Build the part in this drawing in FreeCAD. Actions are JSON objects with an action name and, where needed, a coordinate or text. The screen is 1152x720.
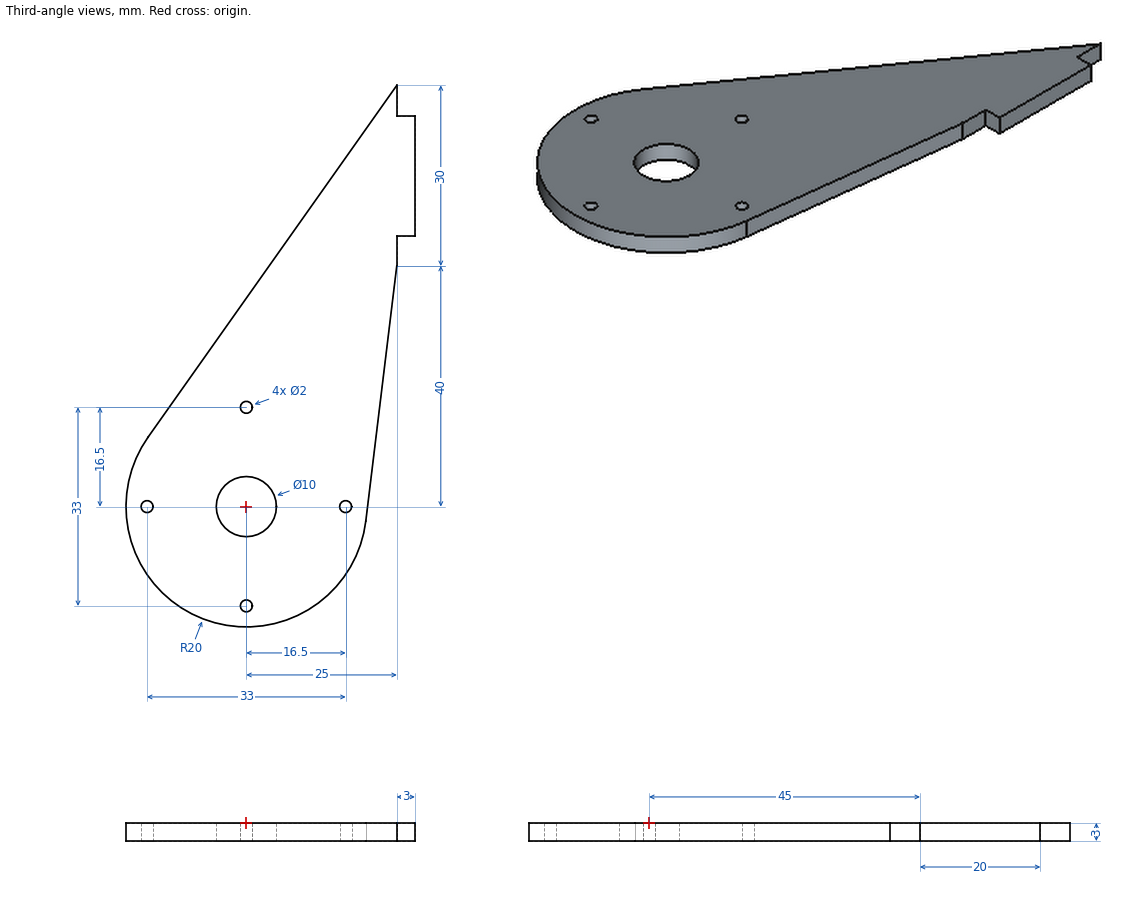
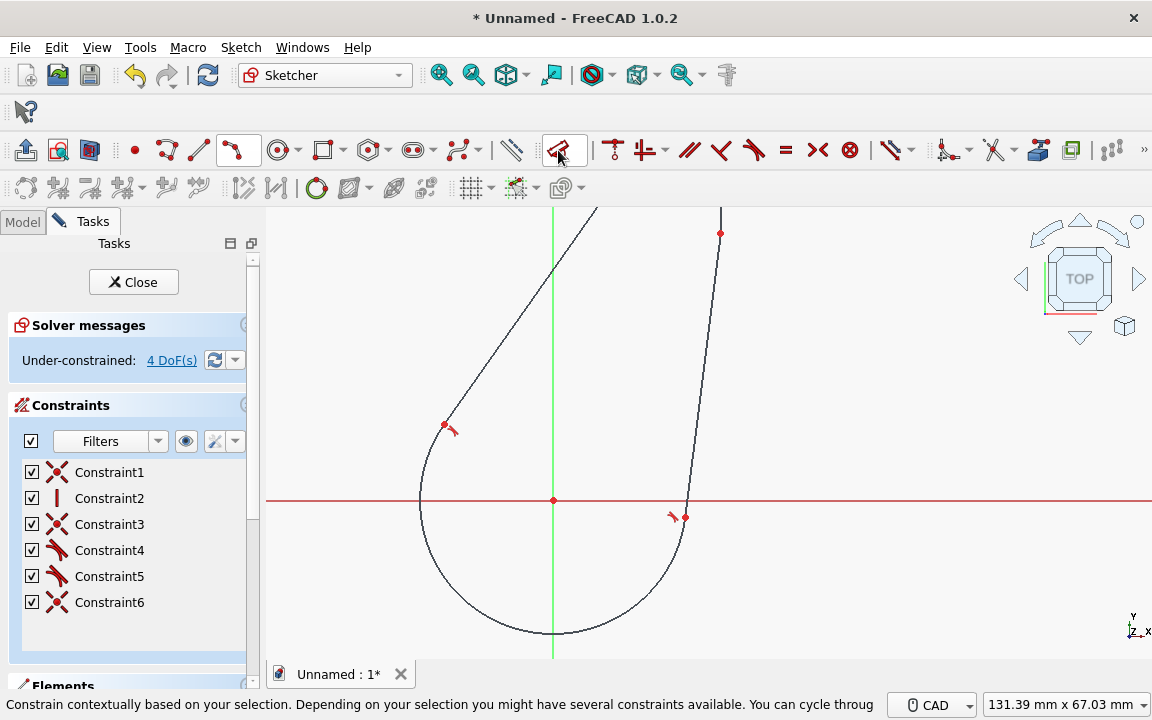
{"action": "left_click", "coordinate": [435, 562]}
{"action": "left_click", "coordinate": [407, 577]}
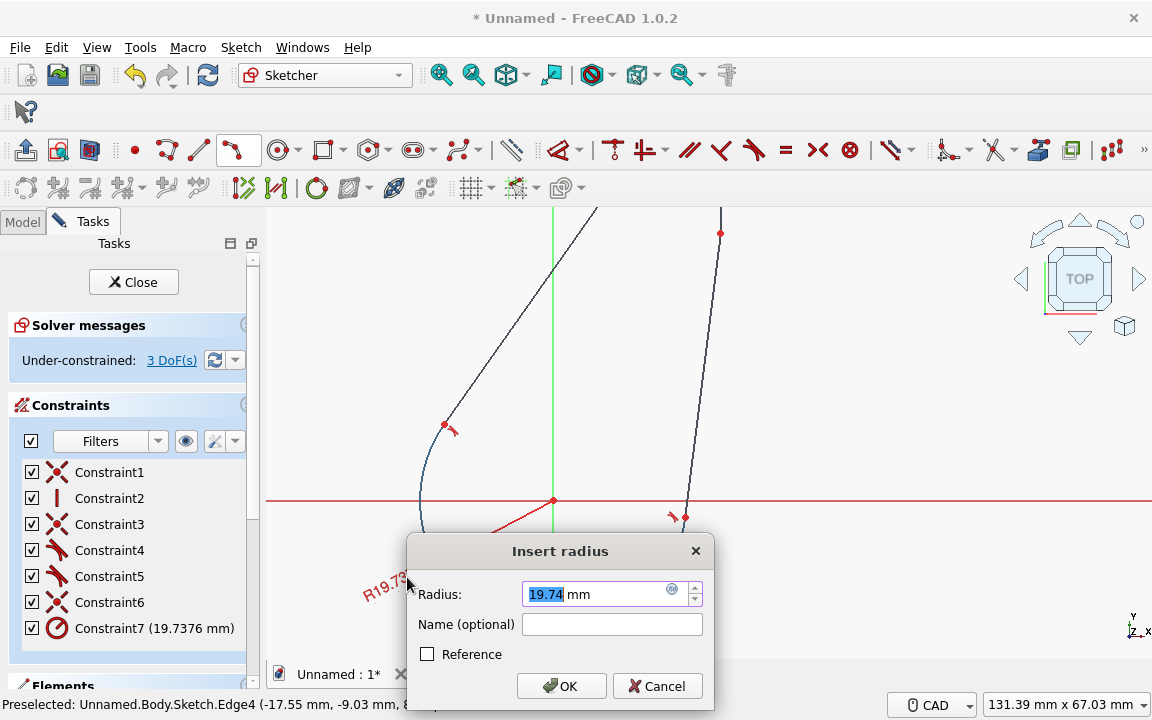
{"action": "type", "text": "20"}
{"action": "key", "text": "Return"}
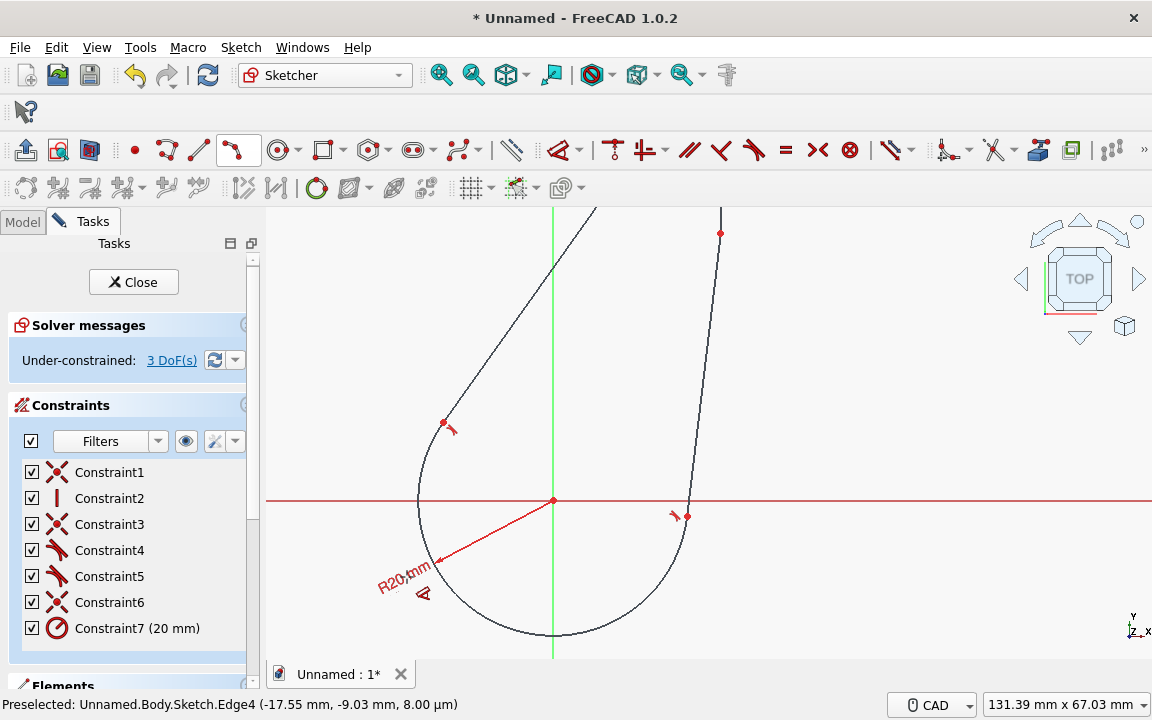
{"action": "scroll", "coordinate": [688, 519], "scroll_direction": "down", "scroll_amount": 4}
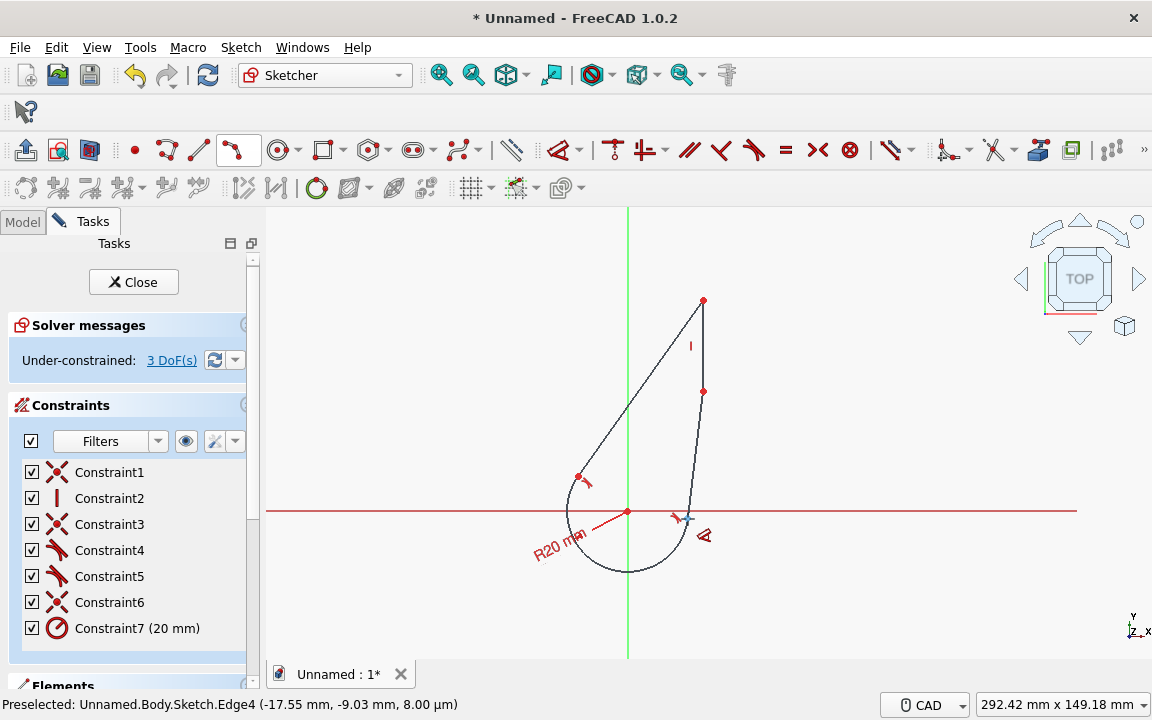
{"action": "left_click", "coordinate": [703, 364]}
{"action": "left_click", "coordinate": [737, 346]}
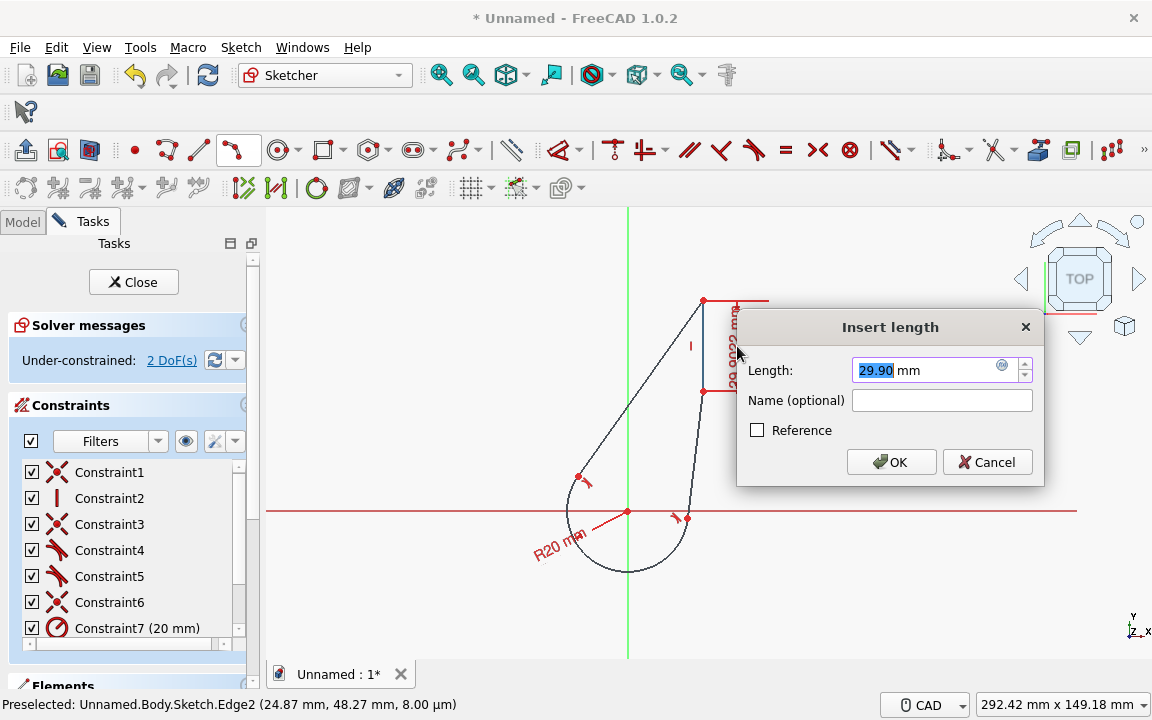
{"action": "type", "text": "30"}
{"action": "key", "text": "Return"}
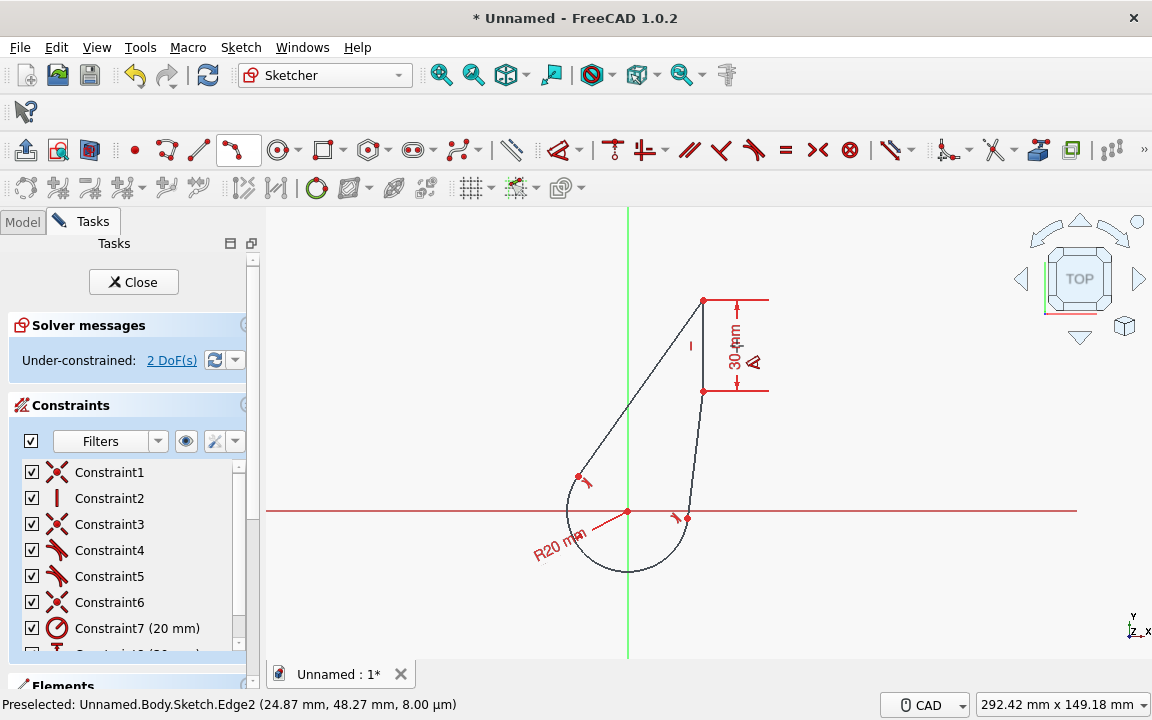
{"action": "left_click", "coordinate": [703, 391]}
{"action": "left_click", "coordinate": [648, 545]}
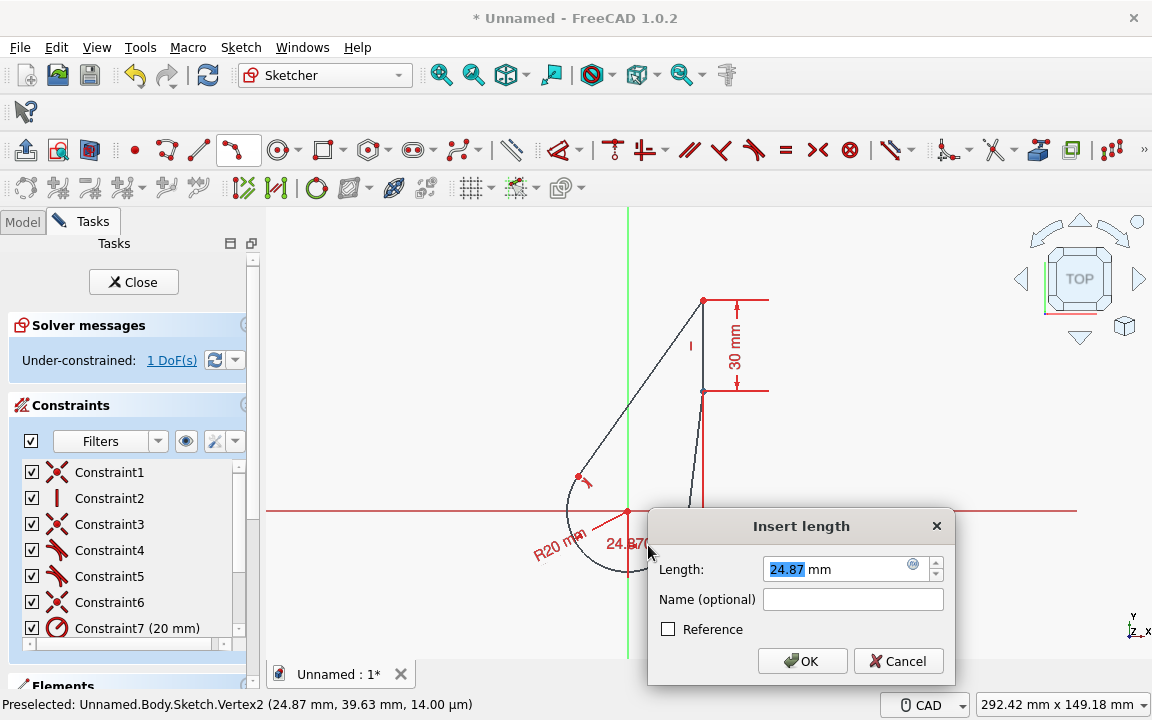
{"action": "type", "text": "25"}
{"action": "key", "text": "Return"}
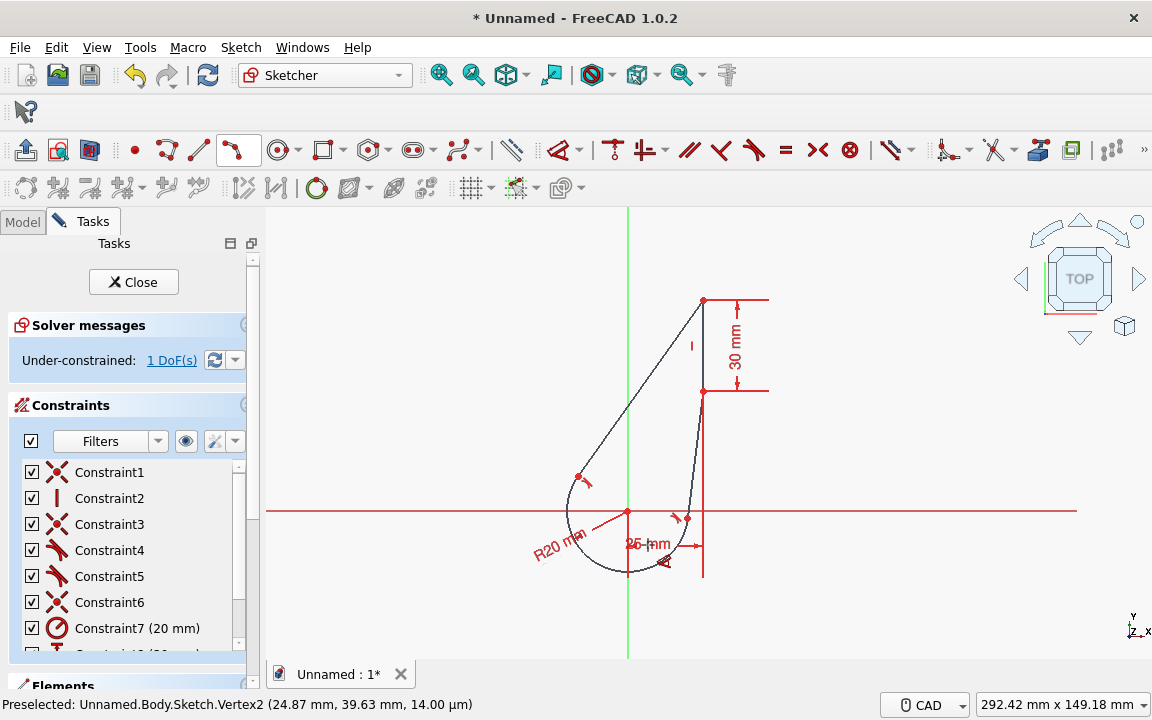
{"action": "left_click", "coordinate": [703, 391]}
{"action": "left_click", "coordinate": [737, 451]}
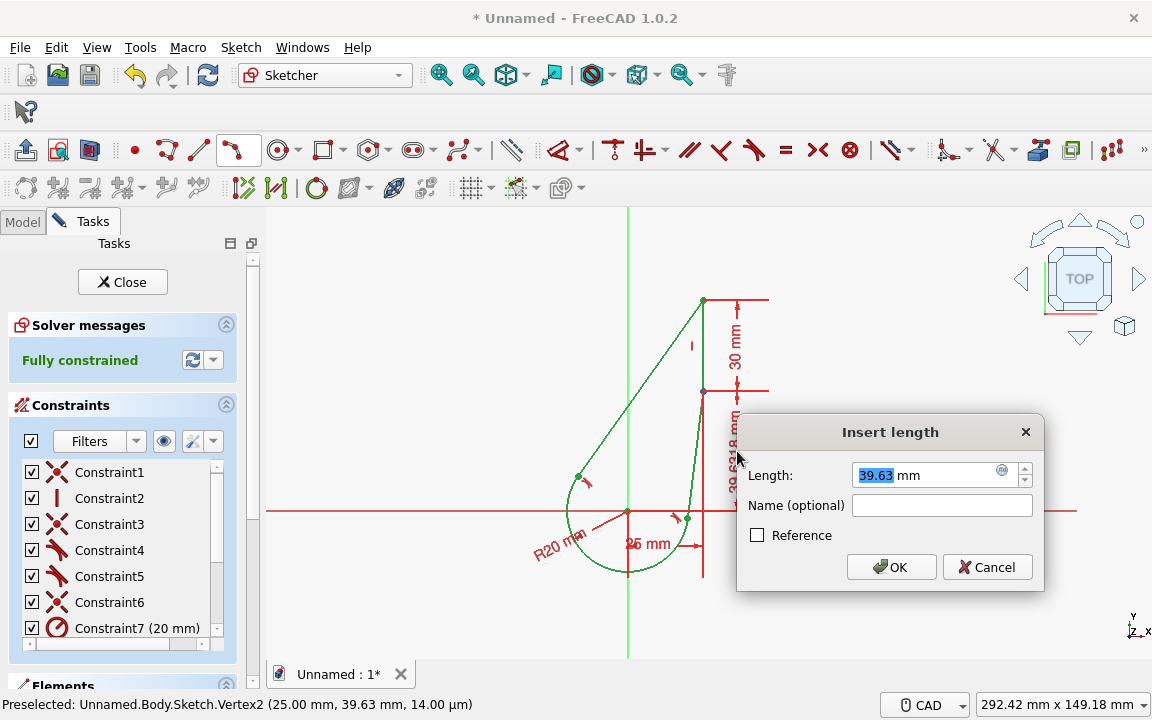
{"action": "type", "text": "40"}
{"action": "key", "text": "Return"}
{"action": "key", "text": "Escape"}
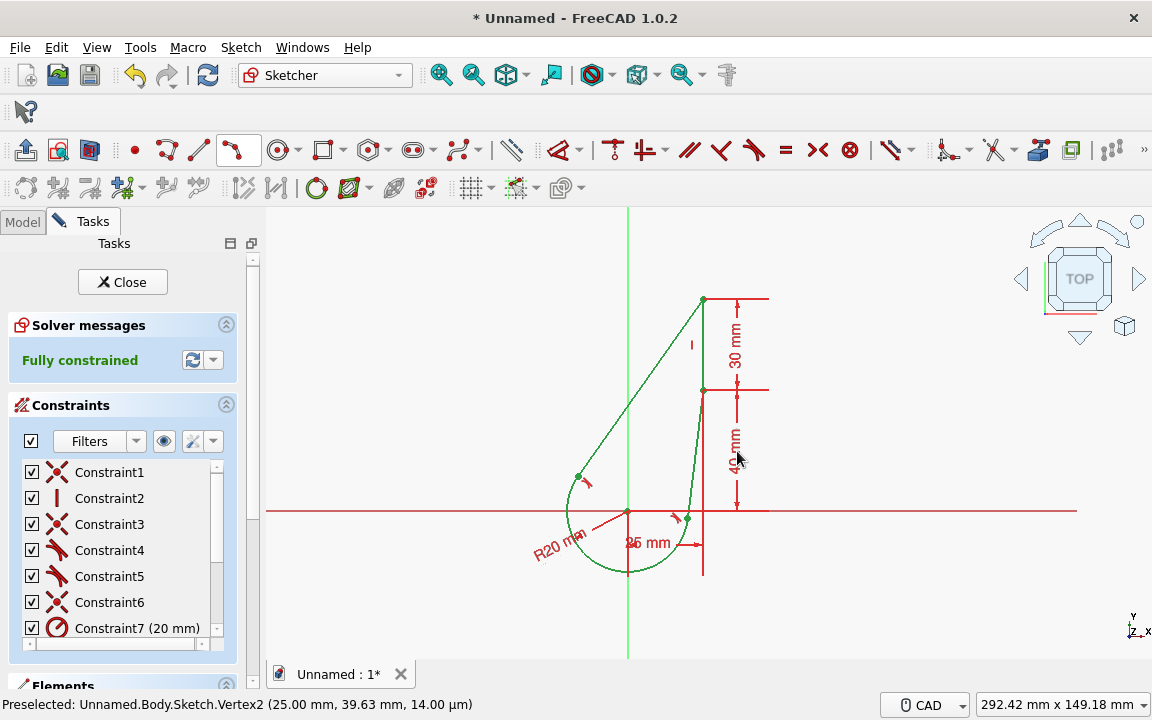
{"action": "left_click", "coordinate": [123, 282]}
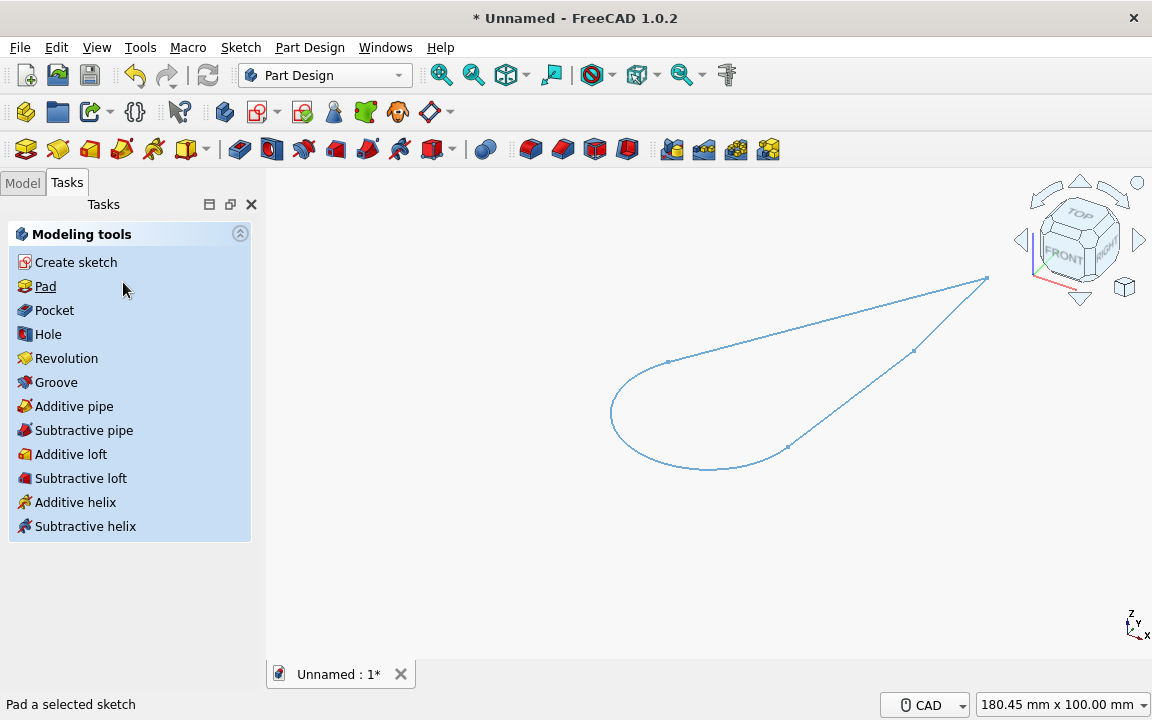
{"action": "left_click", "coordinate": [26, 150]}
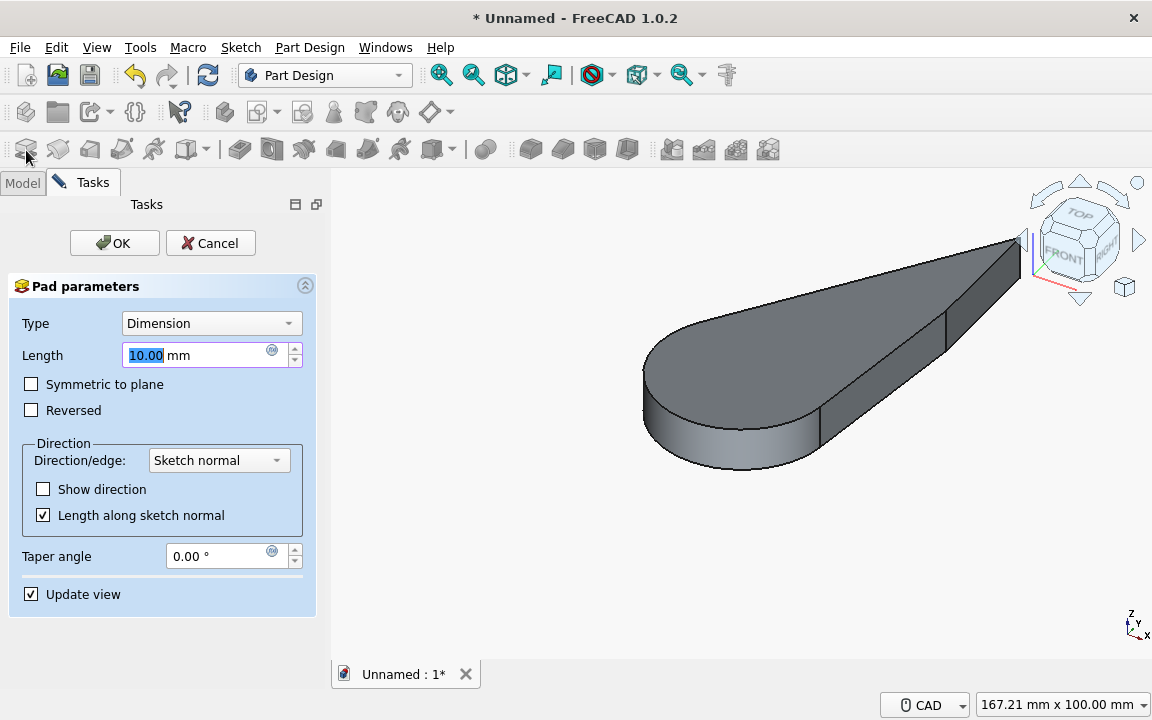
{"action": "type", "text": "3"}
{"action": "key", "text": "Tab"}